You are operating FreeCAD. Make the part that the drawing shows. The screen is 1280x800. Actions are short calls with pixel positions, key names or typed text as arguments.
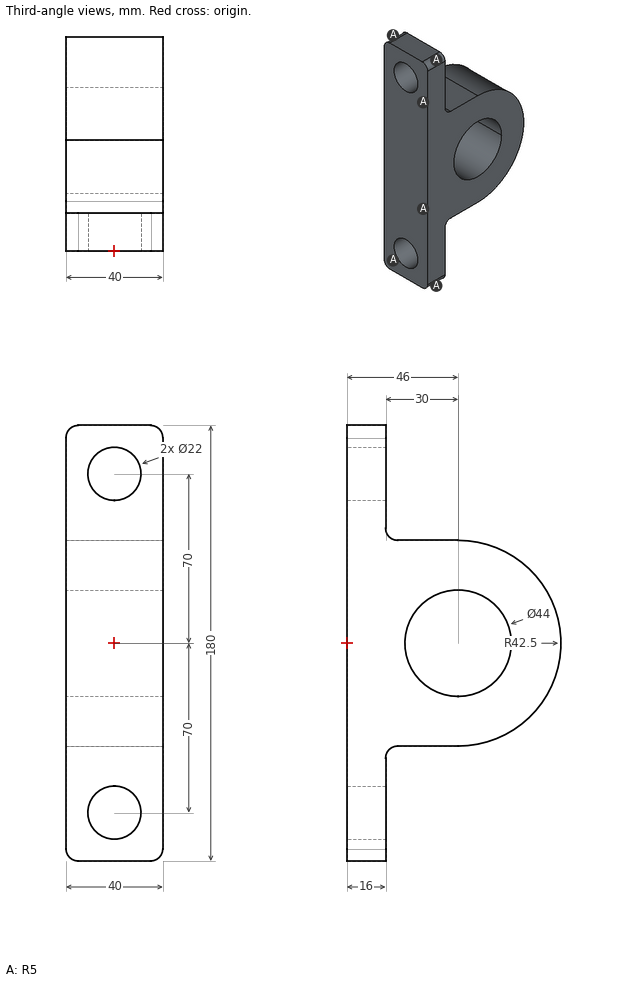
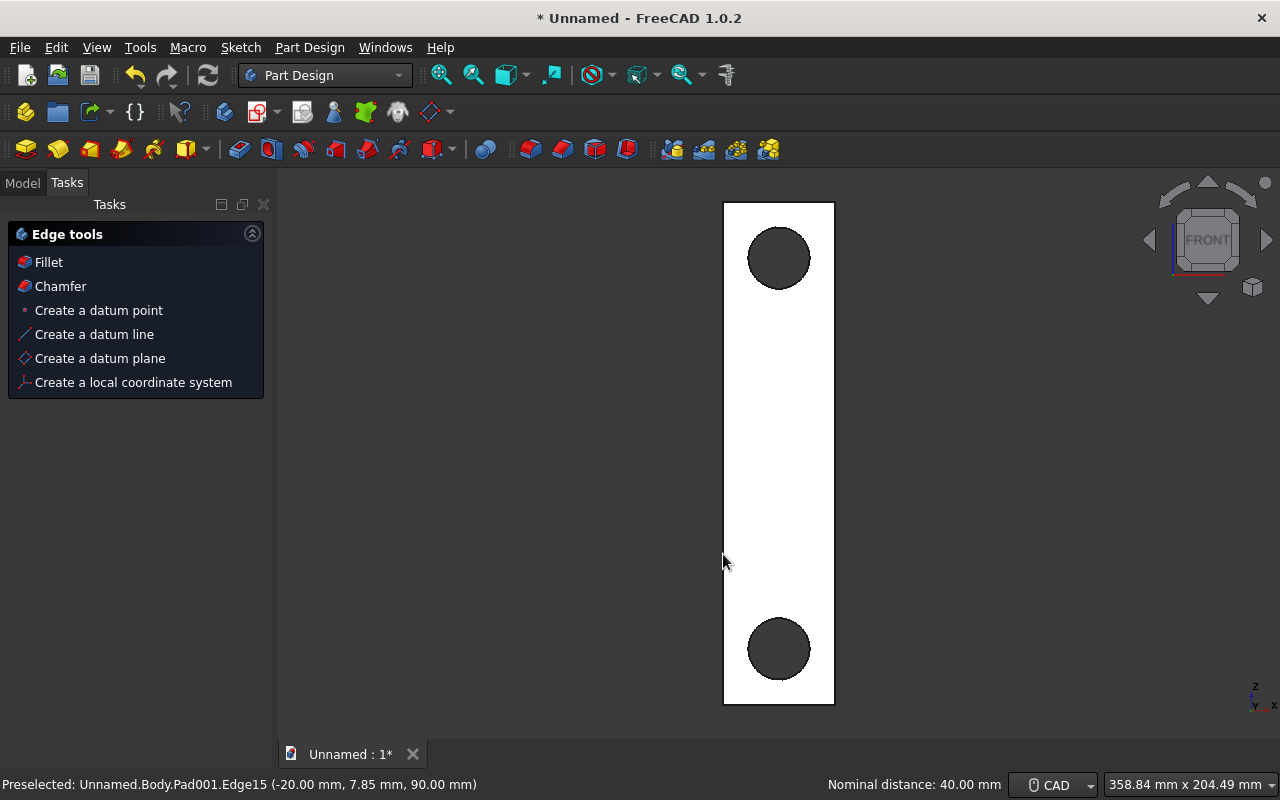
key(3)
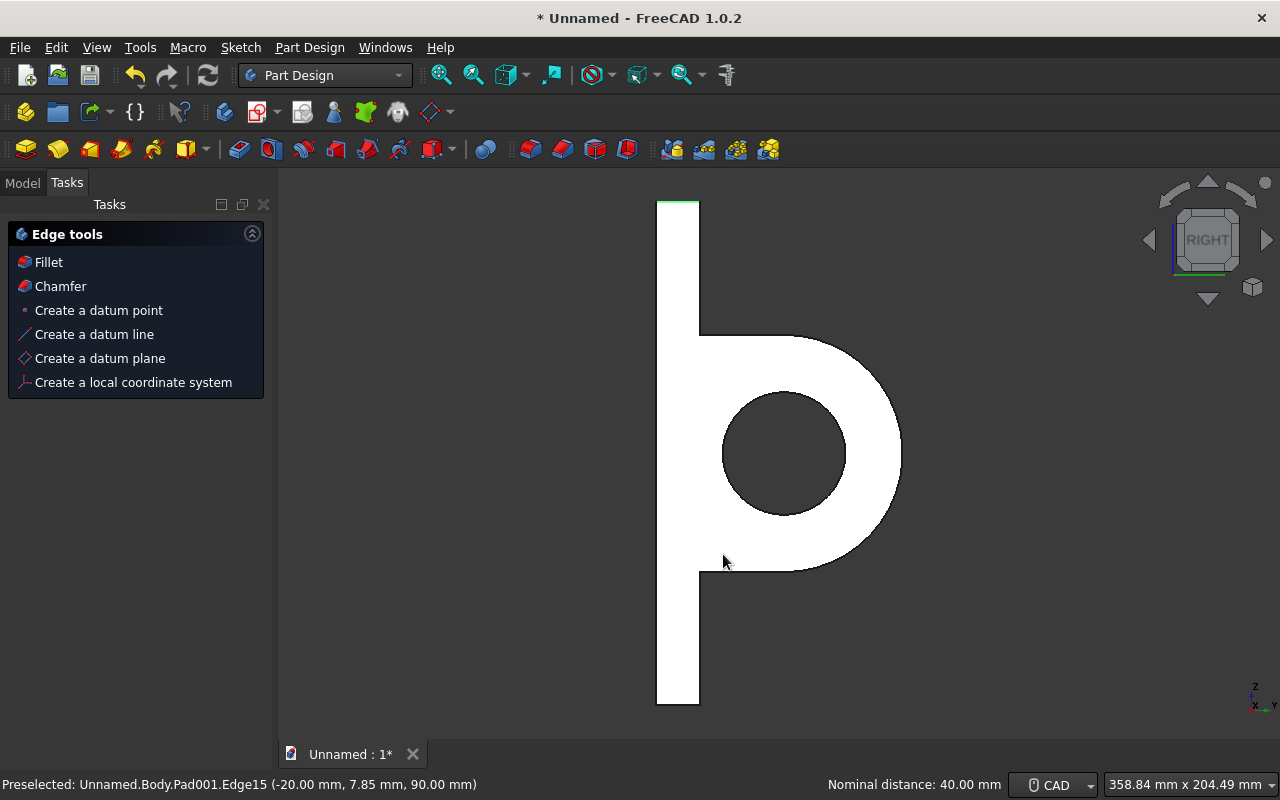
click(678, 704, ctrl)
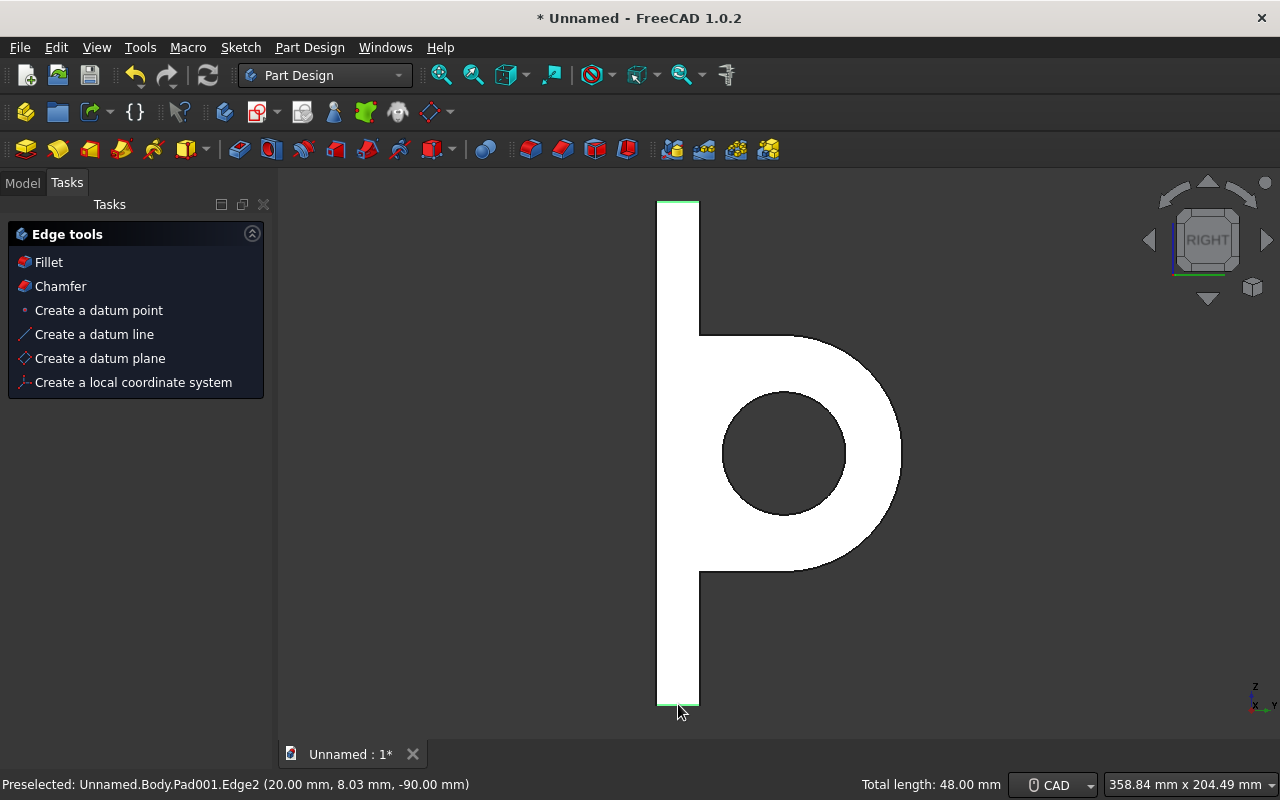
key(5)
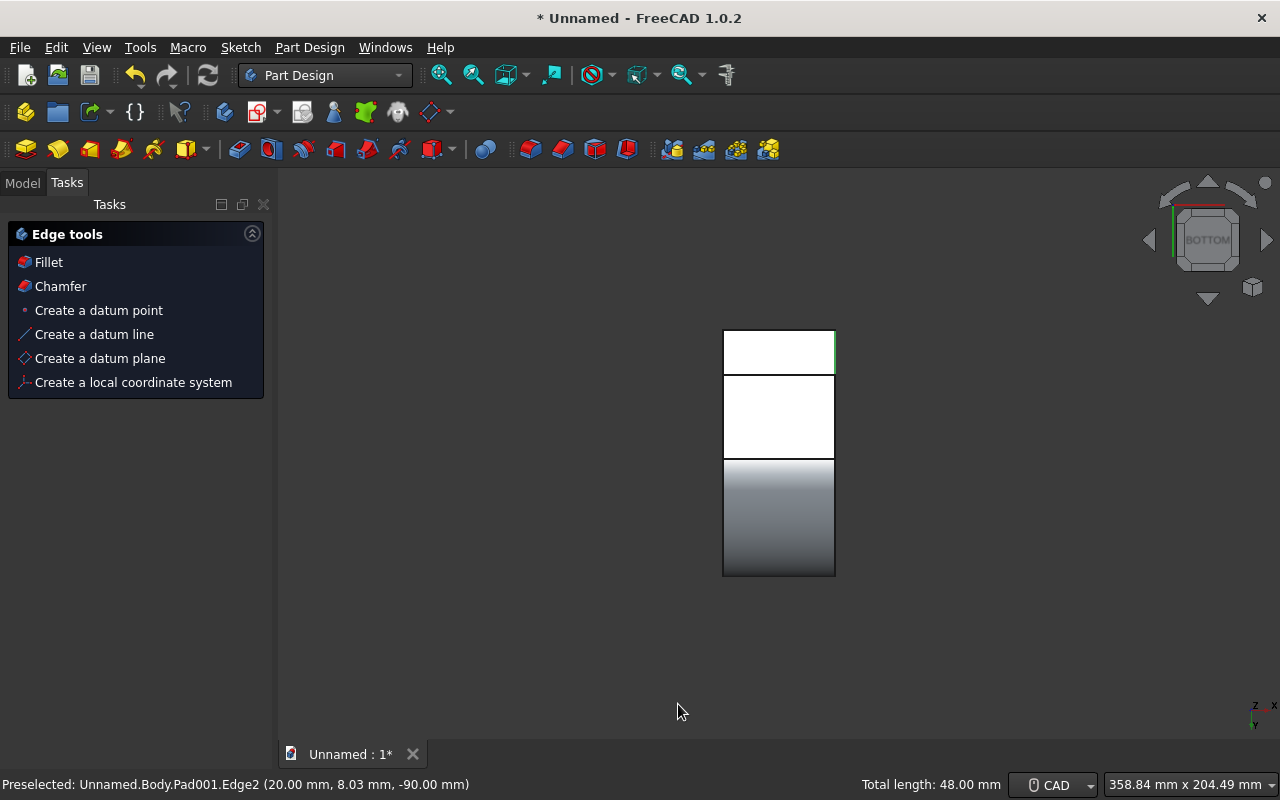
click(442, 76)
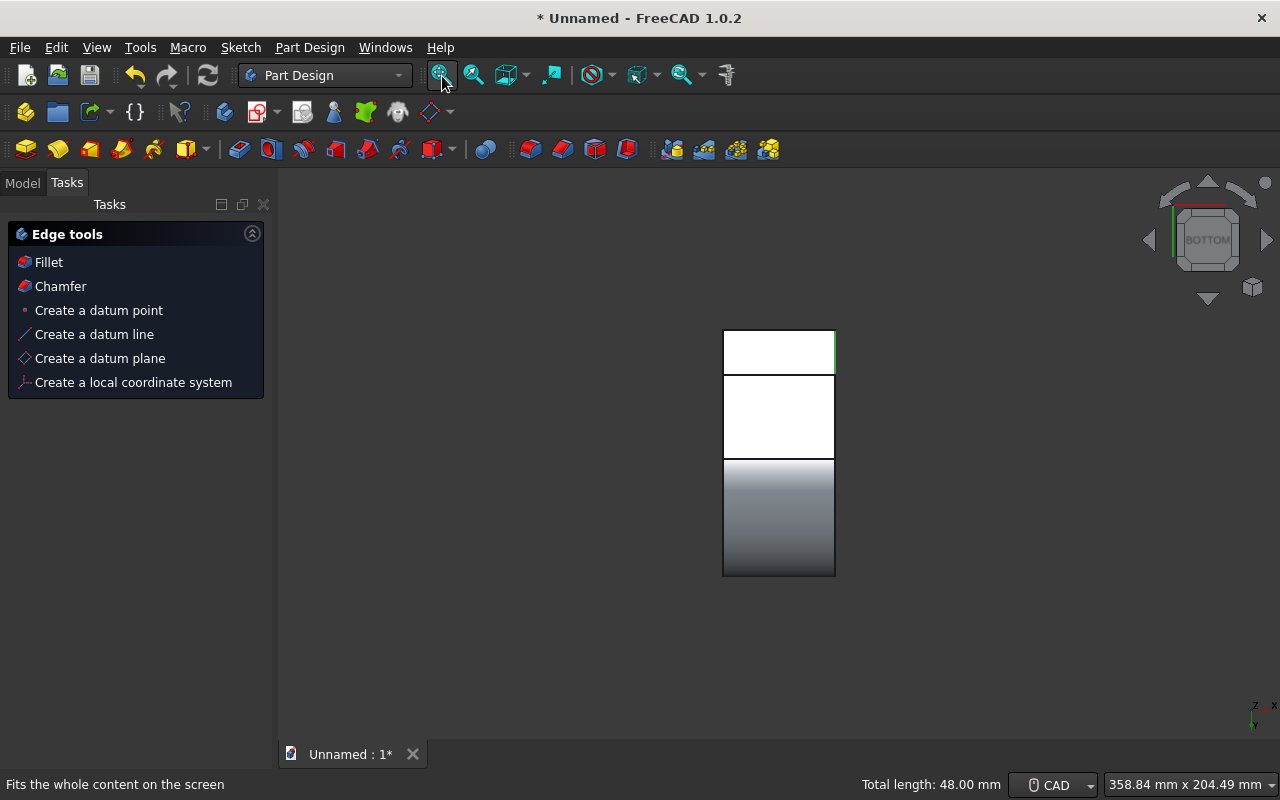
click(723, 351, ctrl)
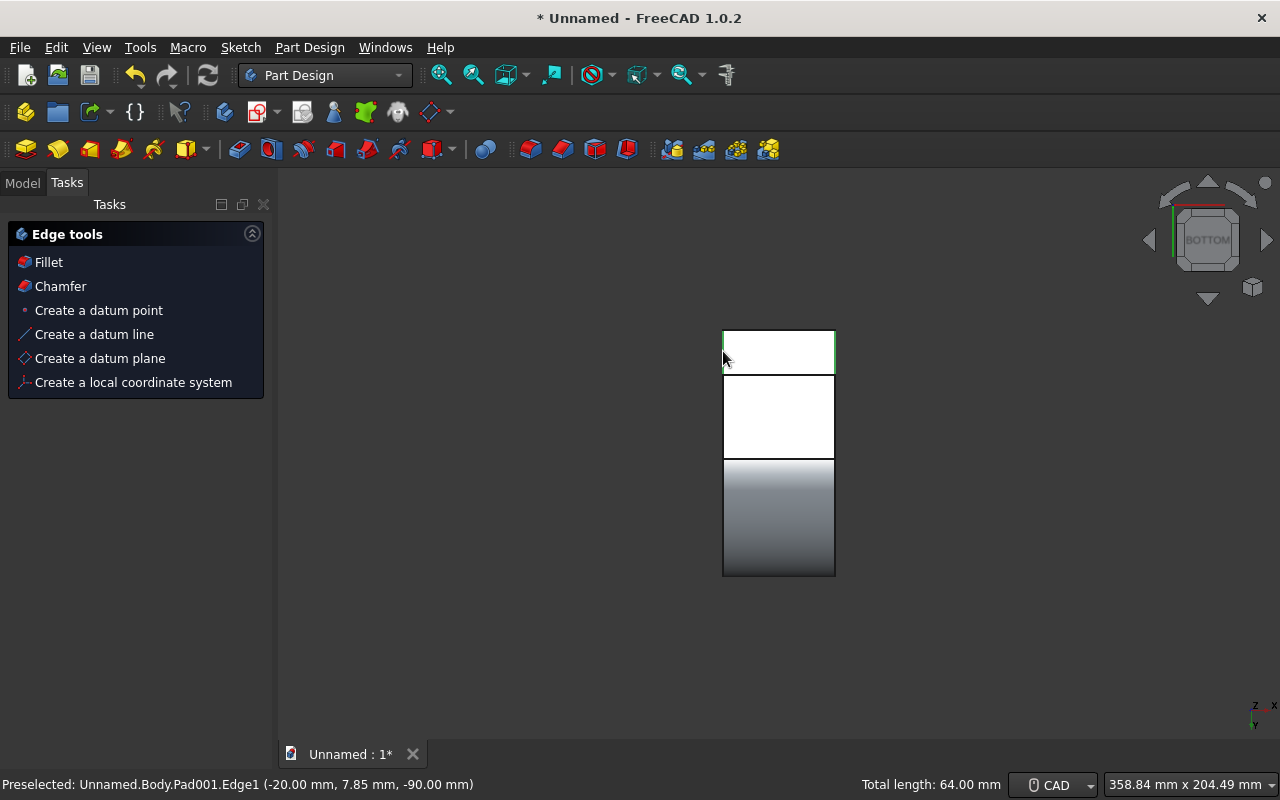
key(4)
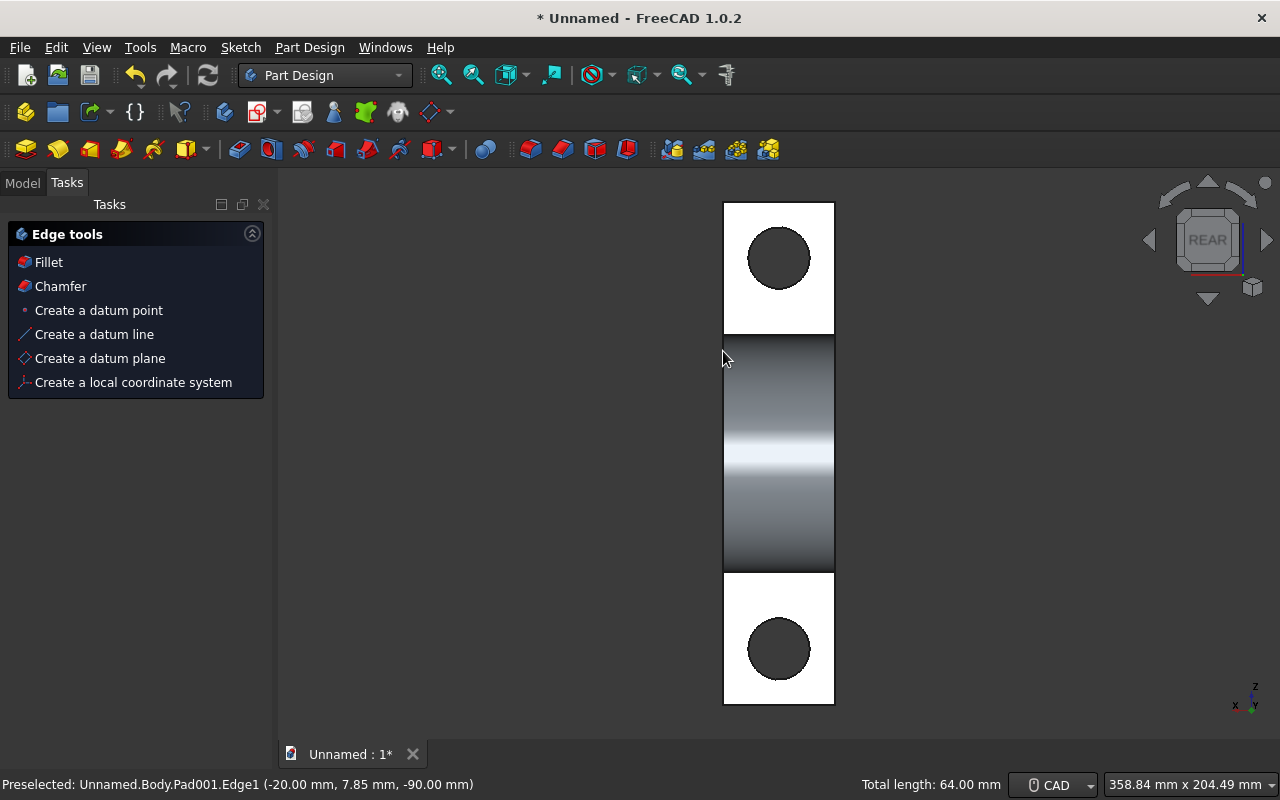
key(6)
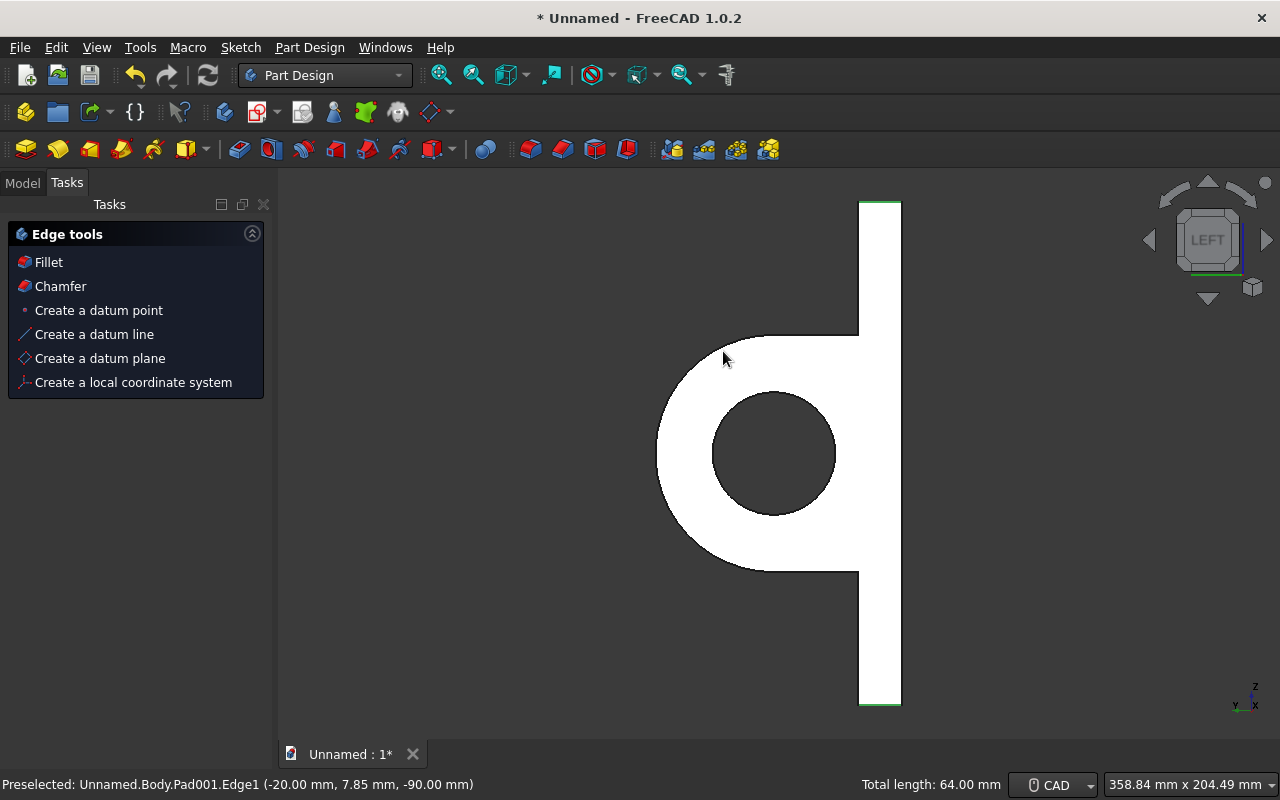
key(v)
key(3)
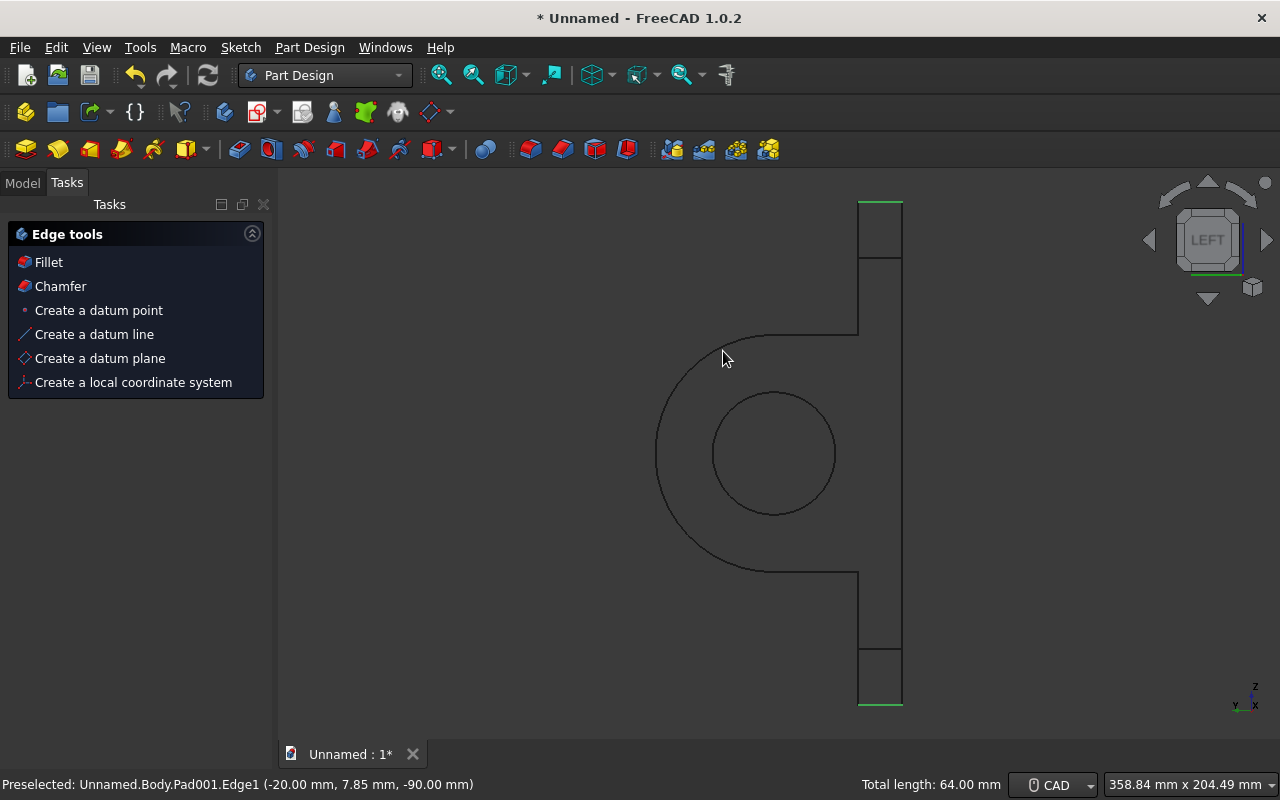
key(0)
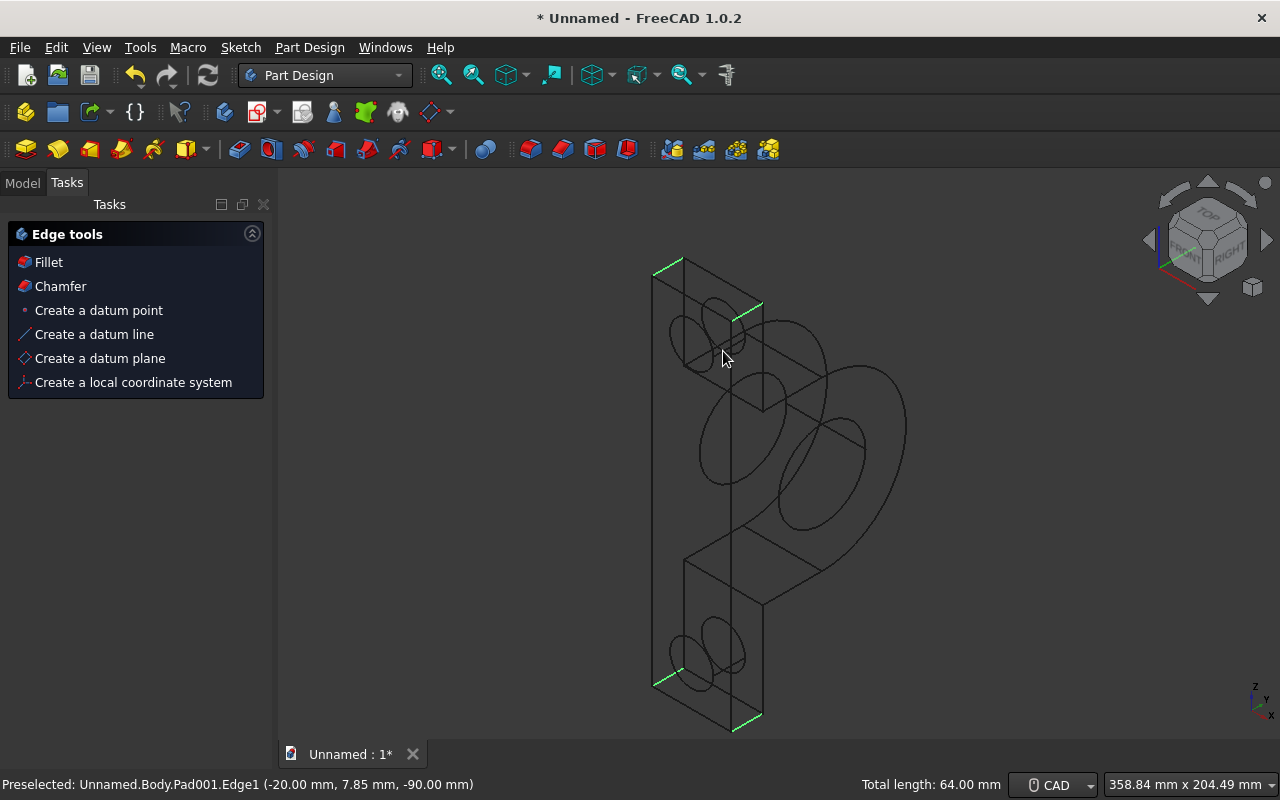
click(723, 388, ctrl)